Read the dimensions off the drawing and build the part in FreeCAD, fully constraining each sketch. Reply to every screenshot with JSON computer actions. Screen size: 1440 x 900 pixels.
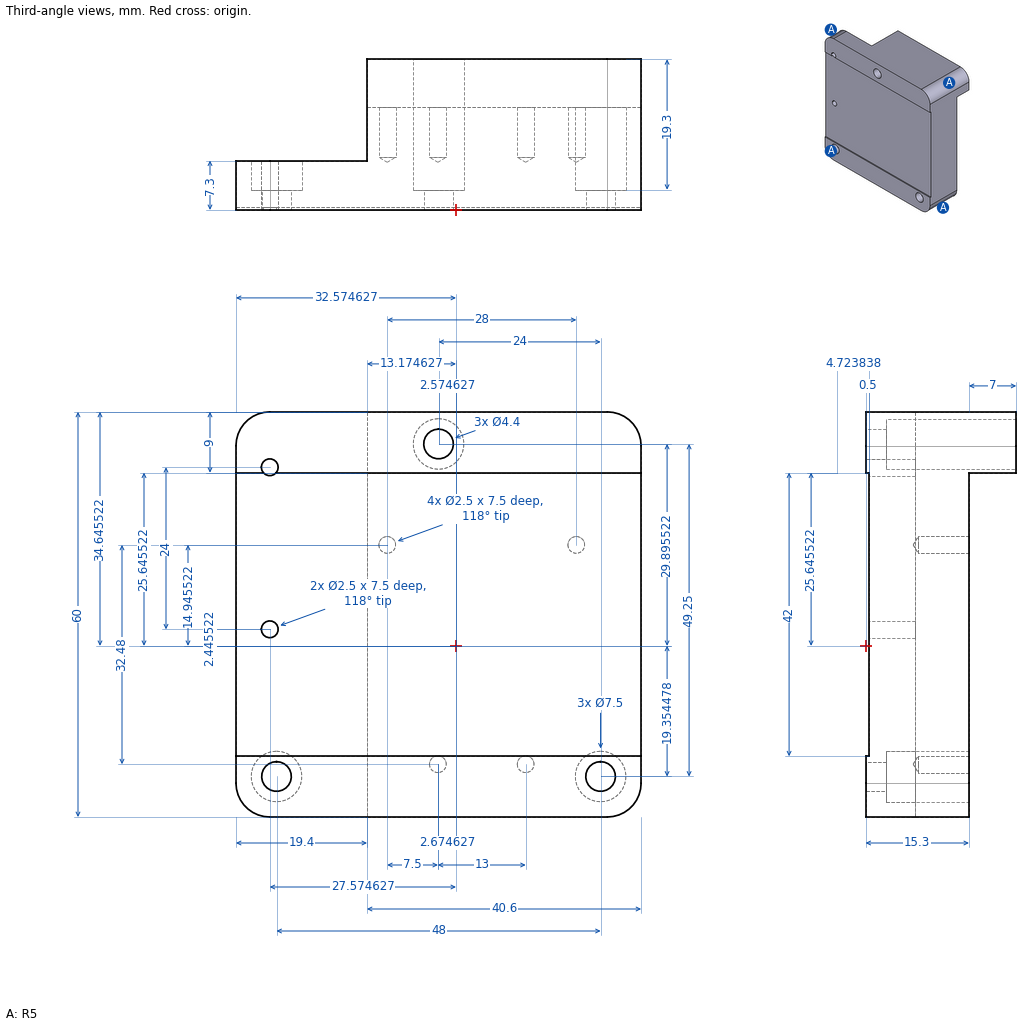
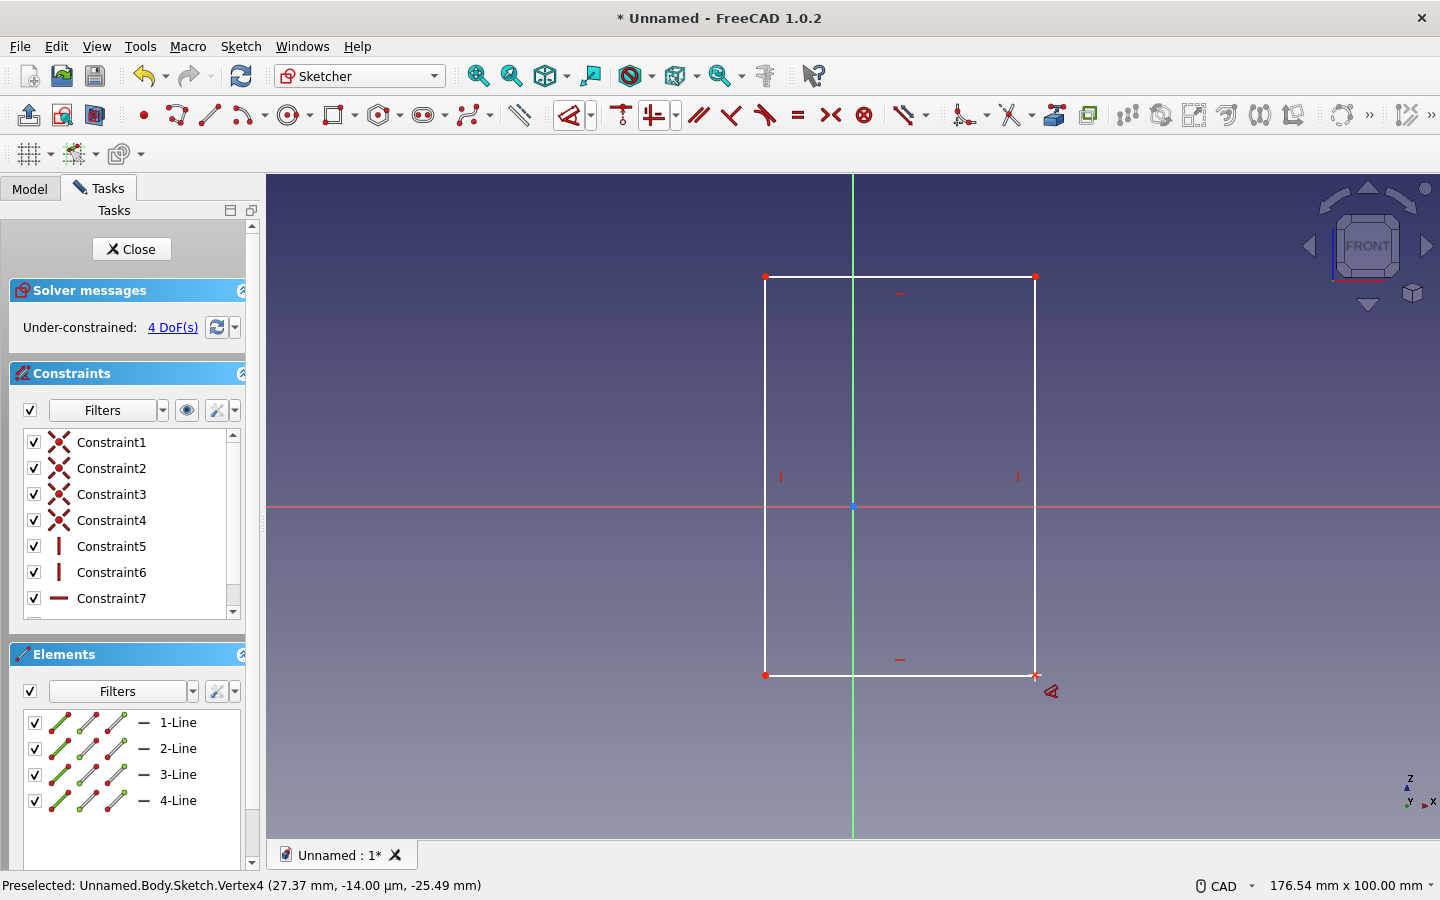
{"action": "left_click", "coordinate": [765, 397]}
{"action": "left_click", "coordinate": [731, 476]}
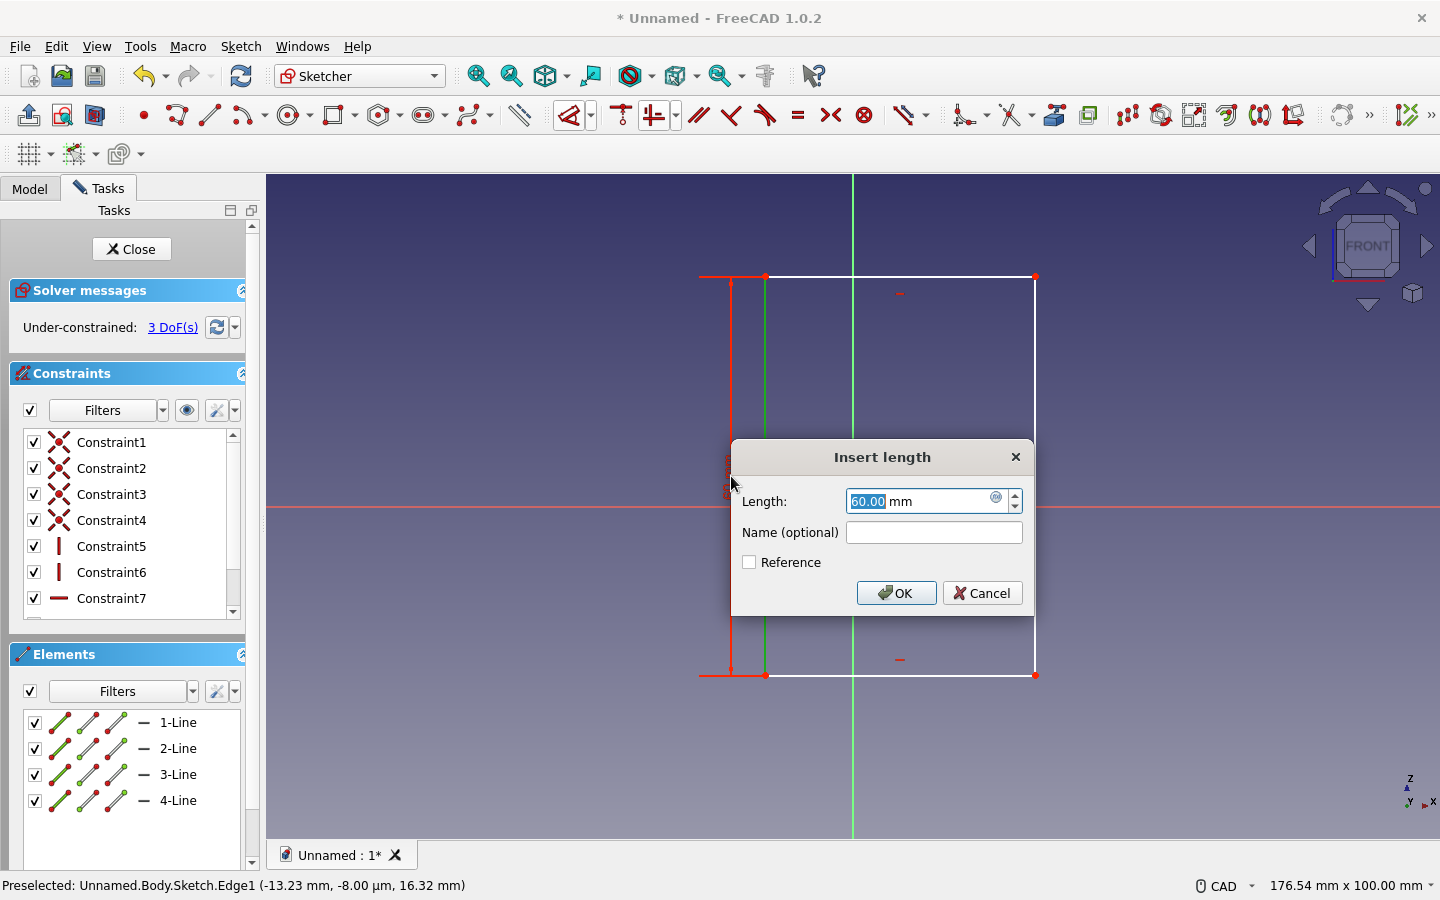
{"action": "type", "text": "60"}
{"action": "key", "text": "Return"}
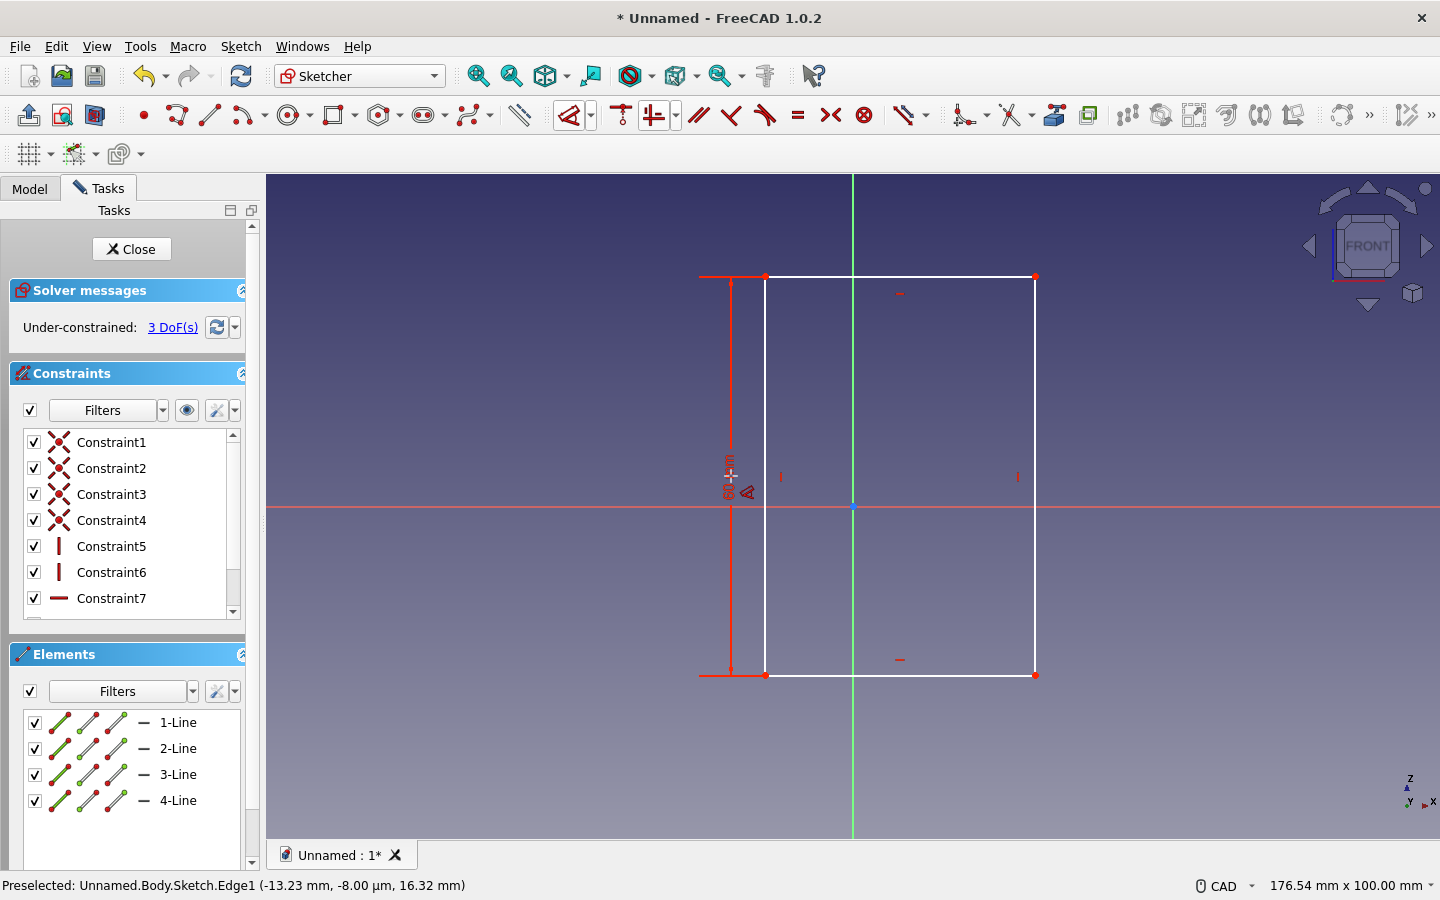
{"action": "left_click", "coordinate": [954, 676]}
{"action": "left_click", "coordinate": [900, 710]}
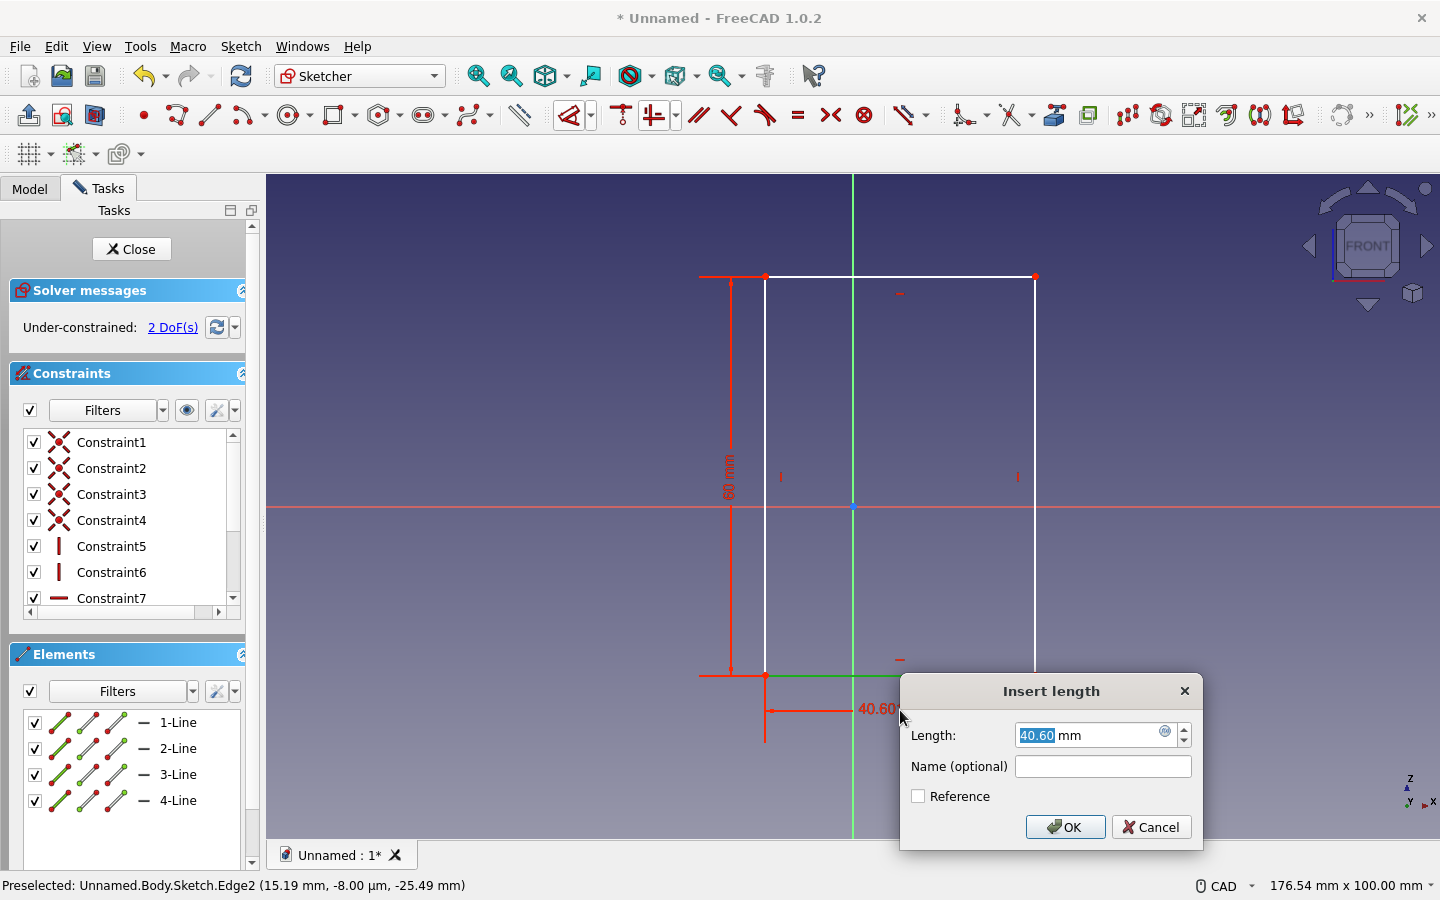
{"action": "type", "text": "40.6"}
{"action": "key", "text": "Return"}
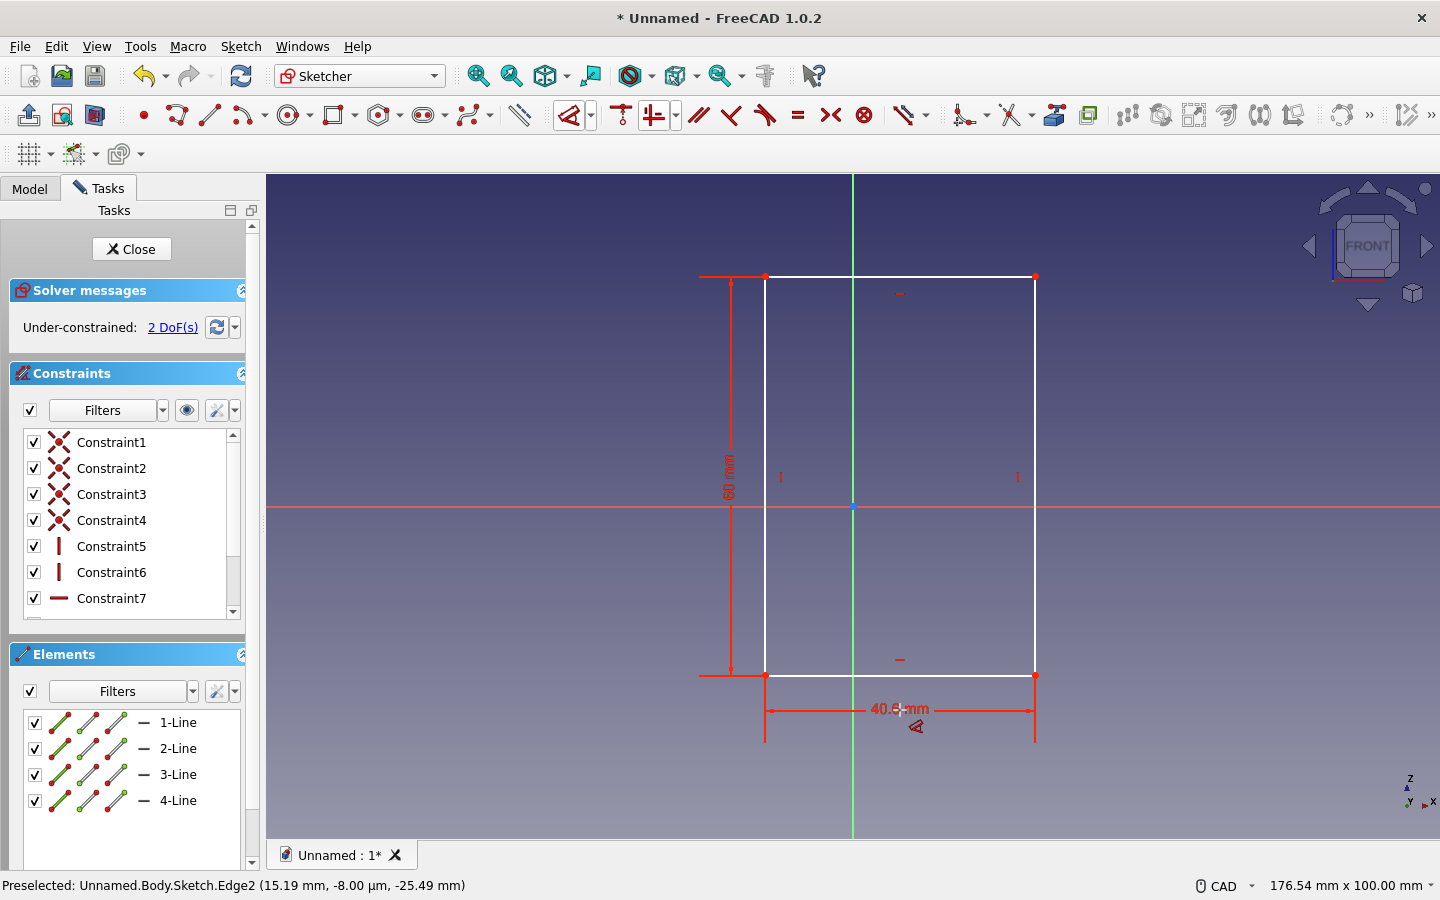
{"action": "left_click", "coordinate": [765, 277]}
{"action": "left_click", "coordinate": [809, 243]}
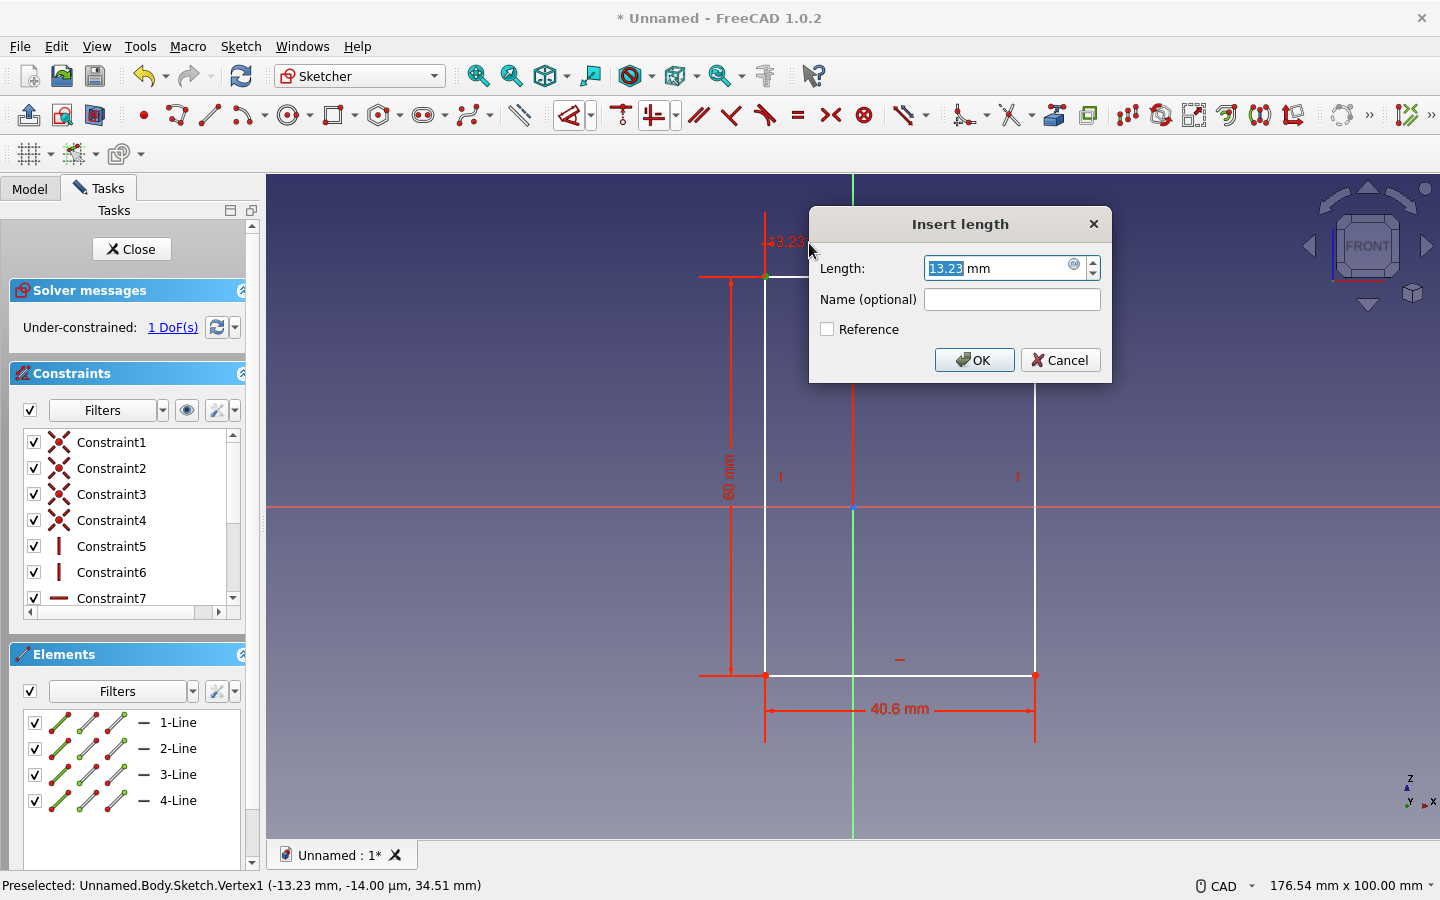
{"action": "type", "text": "13.174627"}
{"action": "key", "text": "Return"}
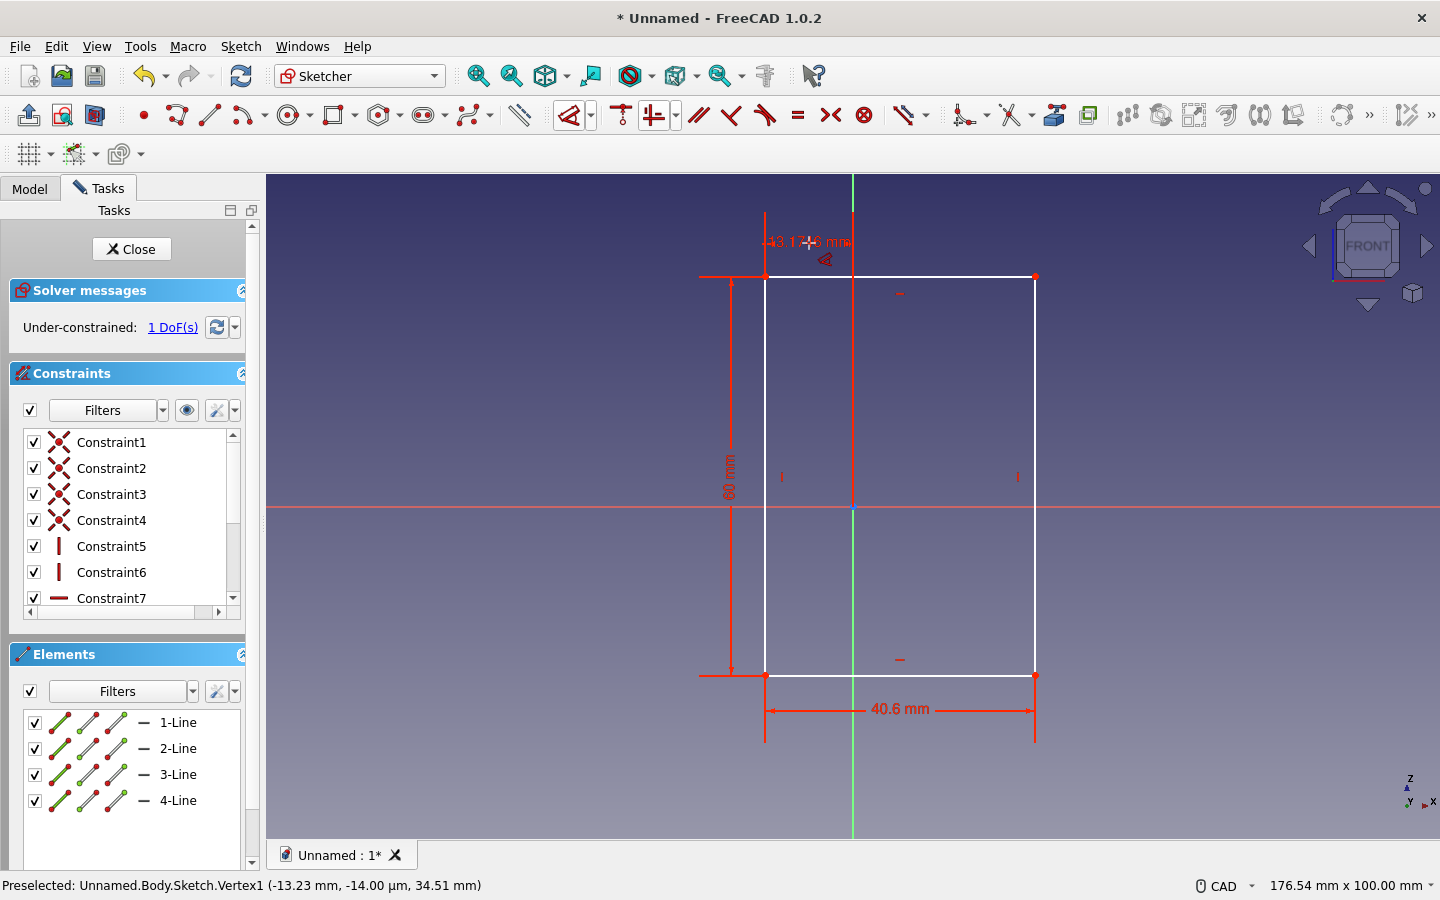
{"action": "left_click", "coordinate": [765, 277]}
{"action": "left_click", "coordinate": [731, 392]}